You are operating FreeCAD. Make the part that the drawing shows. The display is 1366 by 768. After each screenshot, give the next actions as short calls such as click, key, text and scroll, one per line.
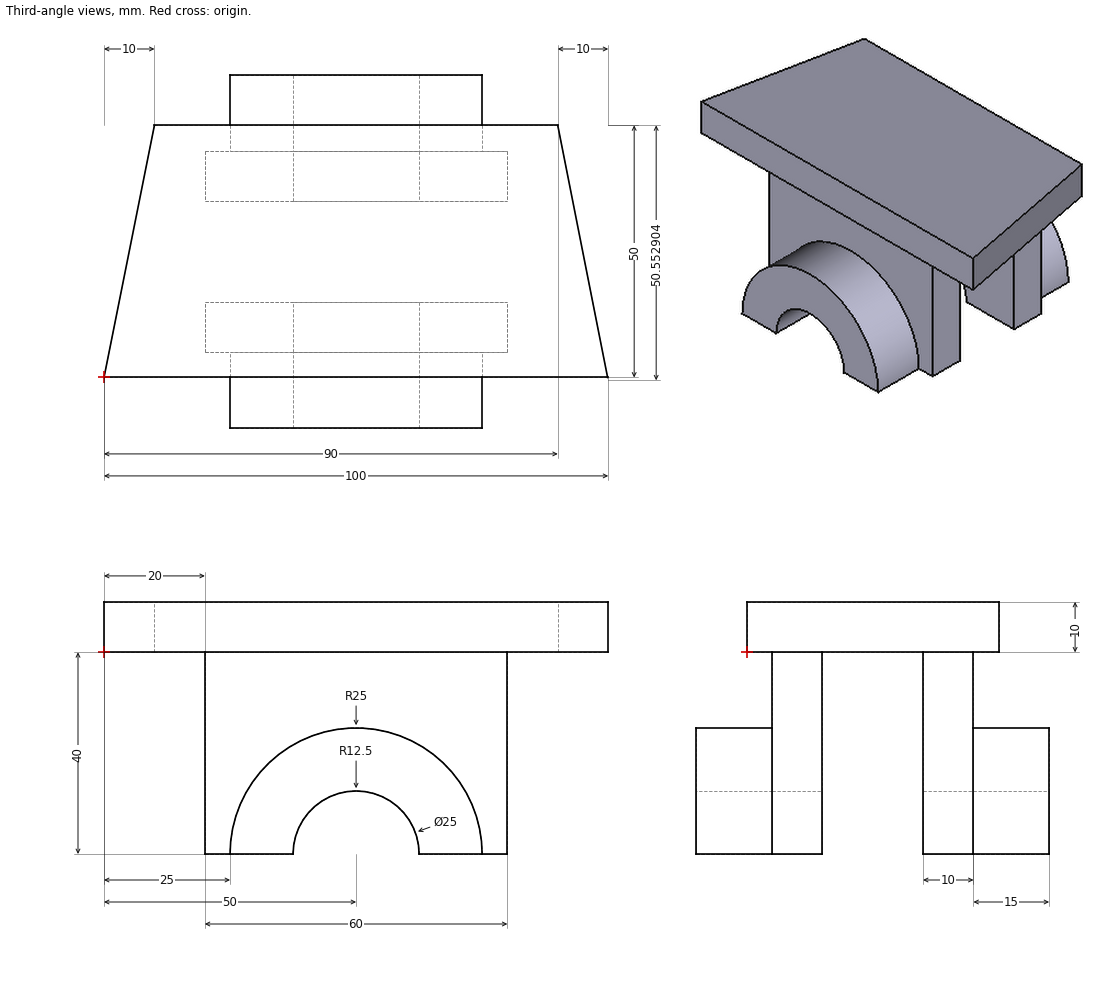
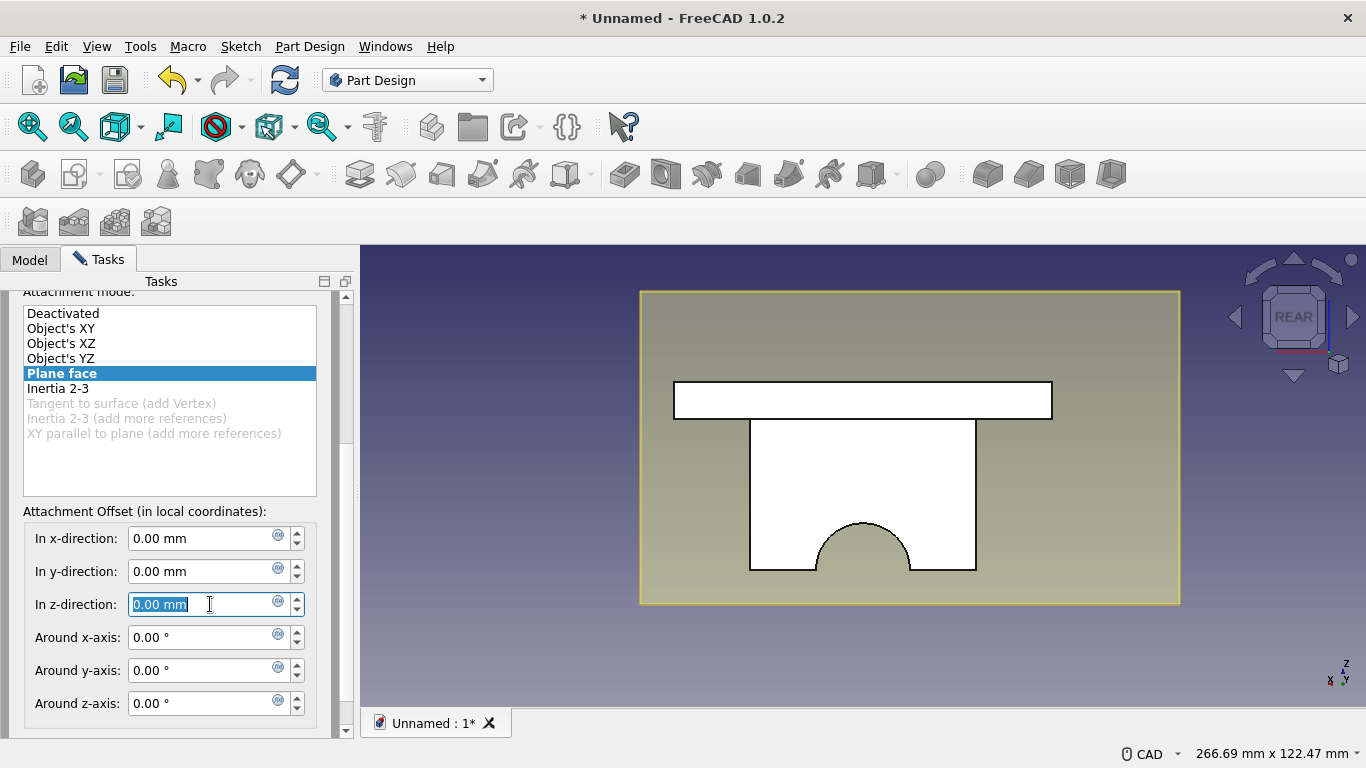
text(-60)
key(Tab)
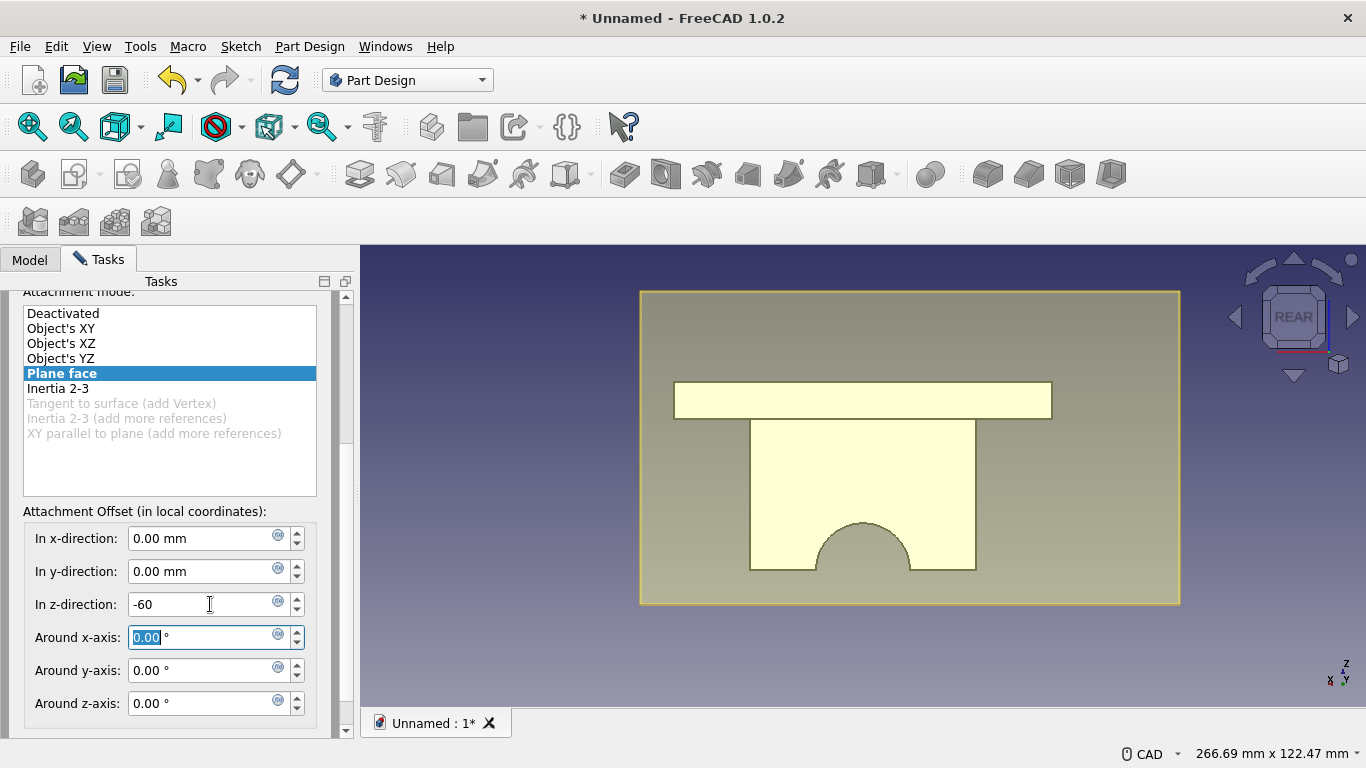
scroll(346, 514, up, 5)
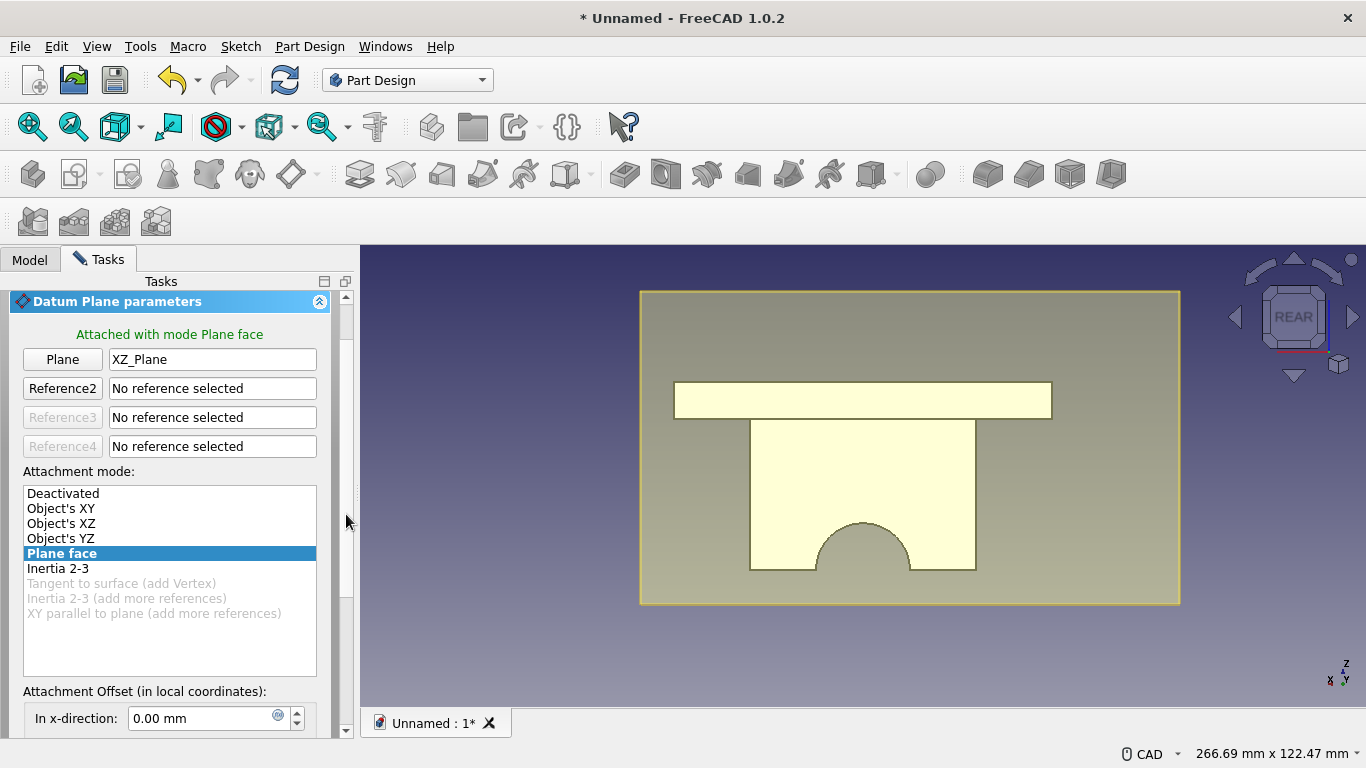
click(127, 320)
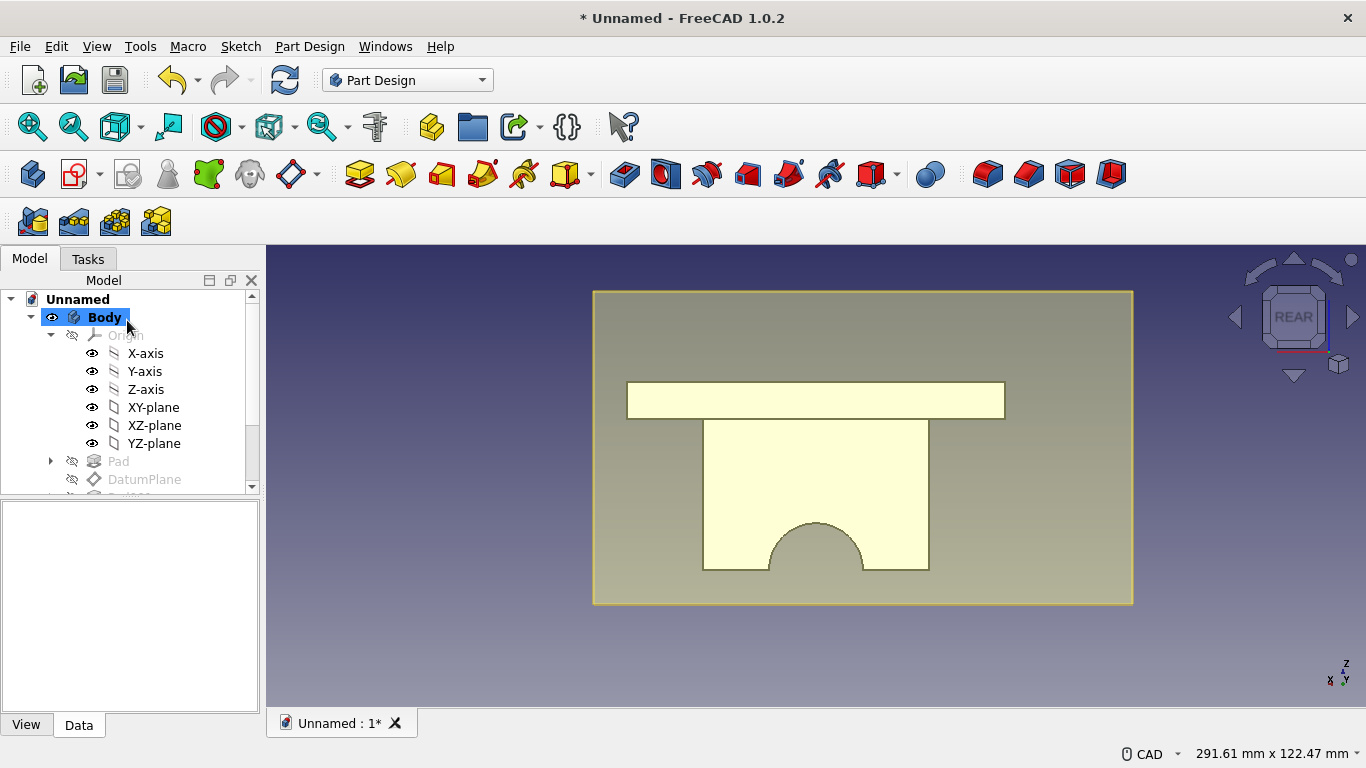
scroll(101, 385, down, 3)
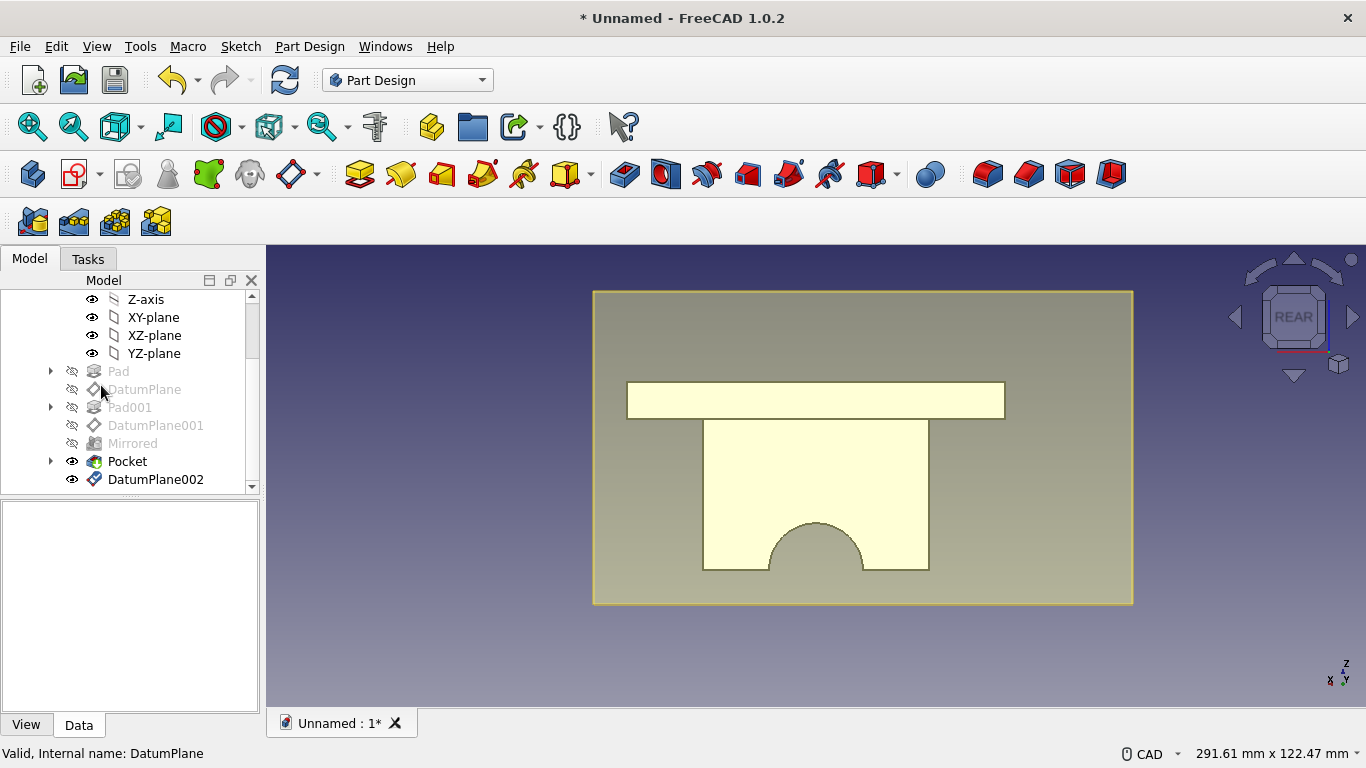
click(117, 479)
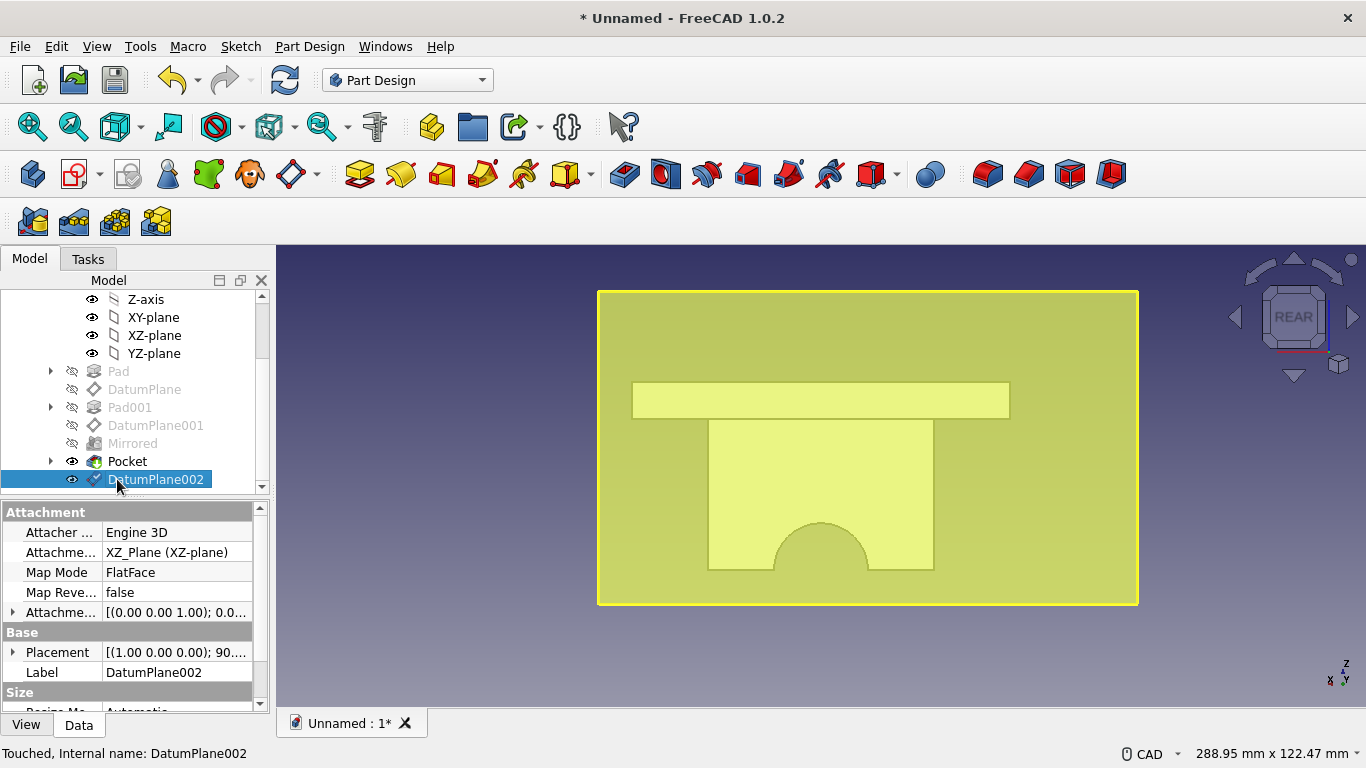
click(74, 174)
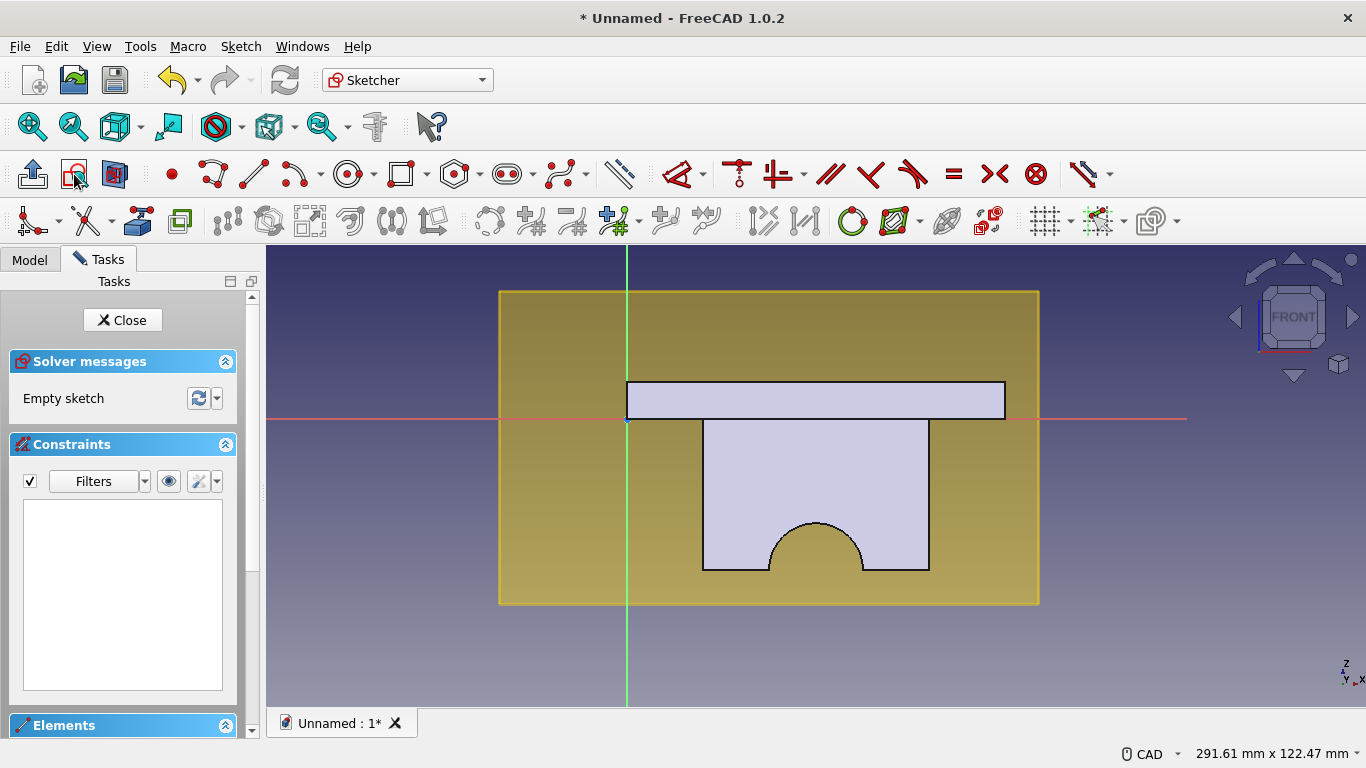
key(q)
key(s)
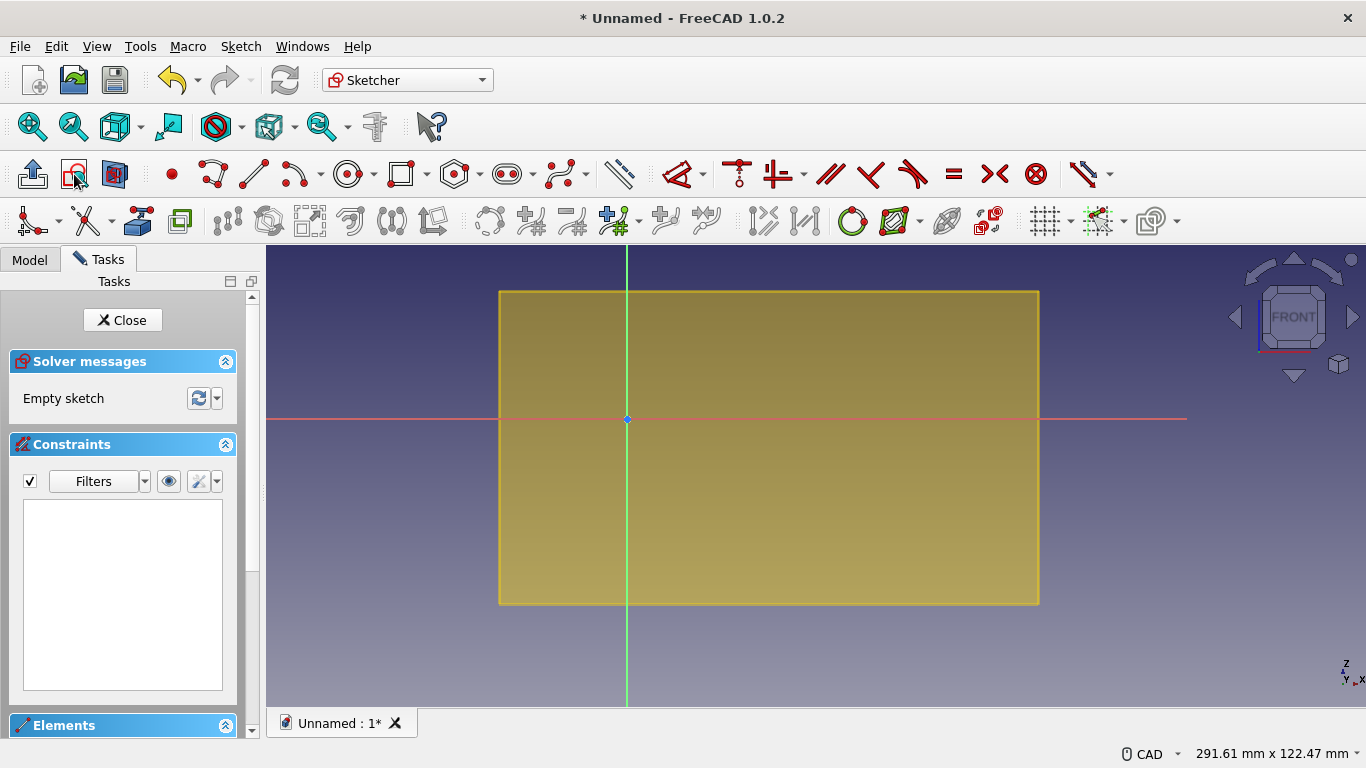
scroll(795, 518, up, 3)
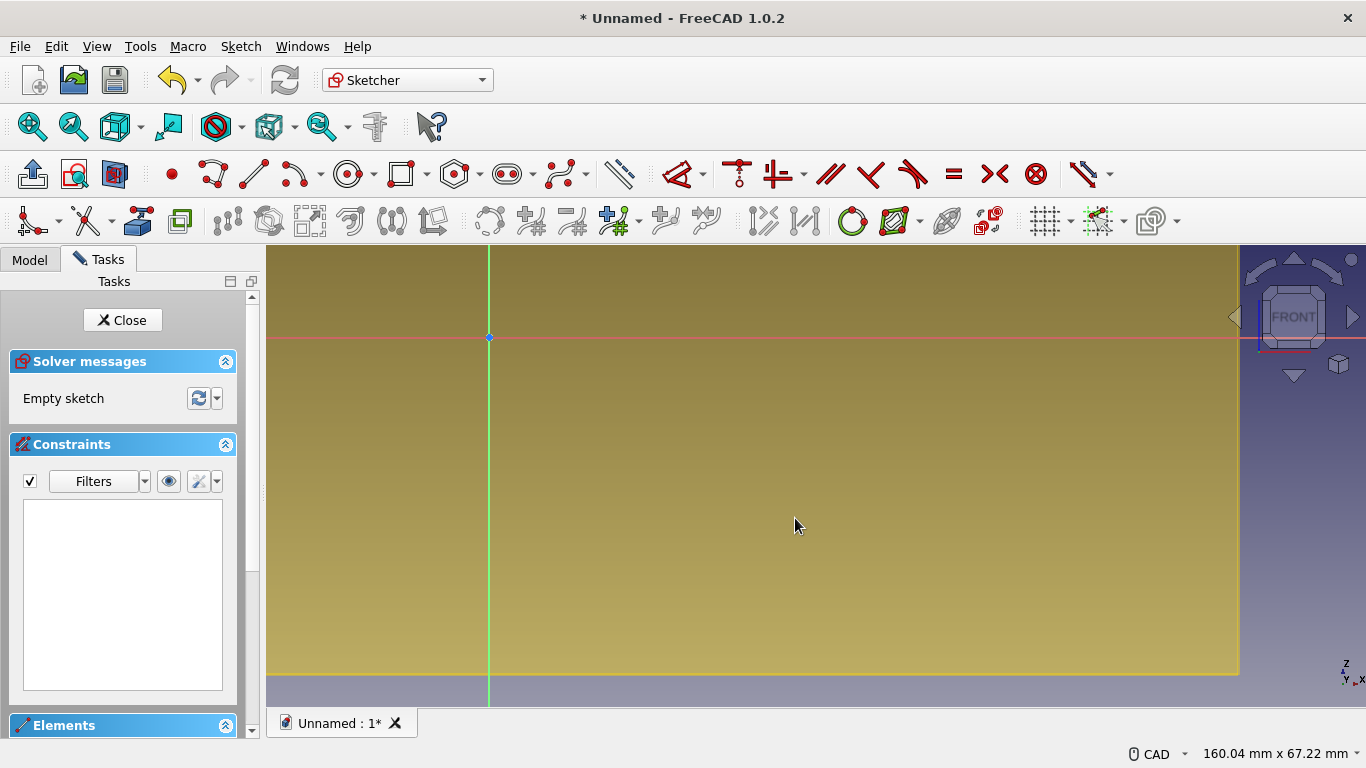
key(g)
key(l)